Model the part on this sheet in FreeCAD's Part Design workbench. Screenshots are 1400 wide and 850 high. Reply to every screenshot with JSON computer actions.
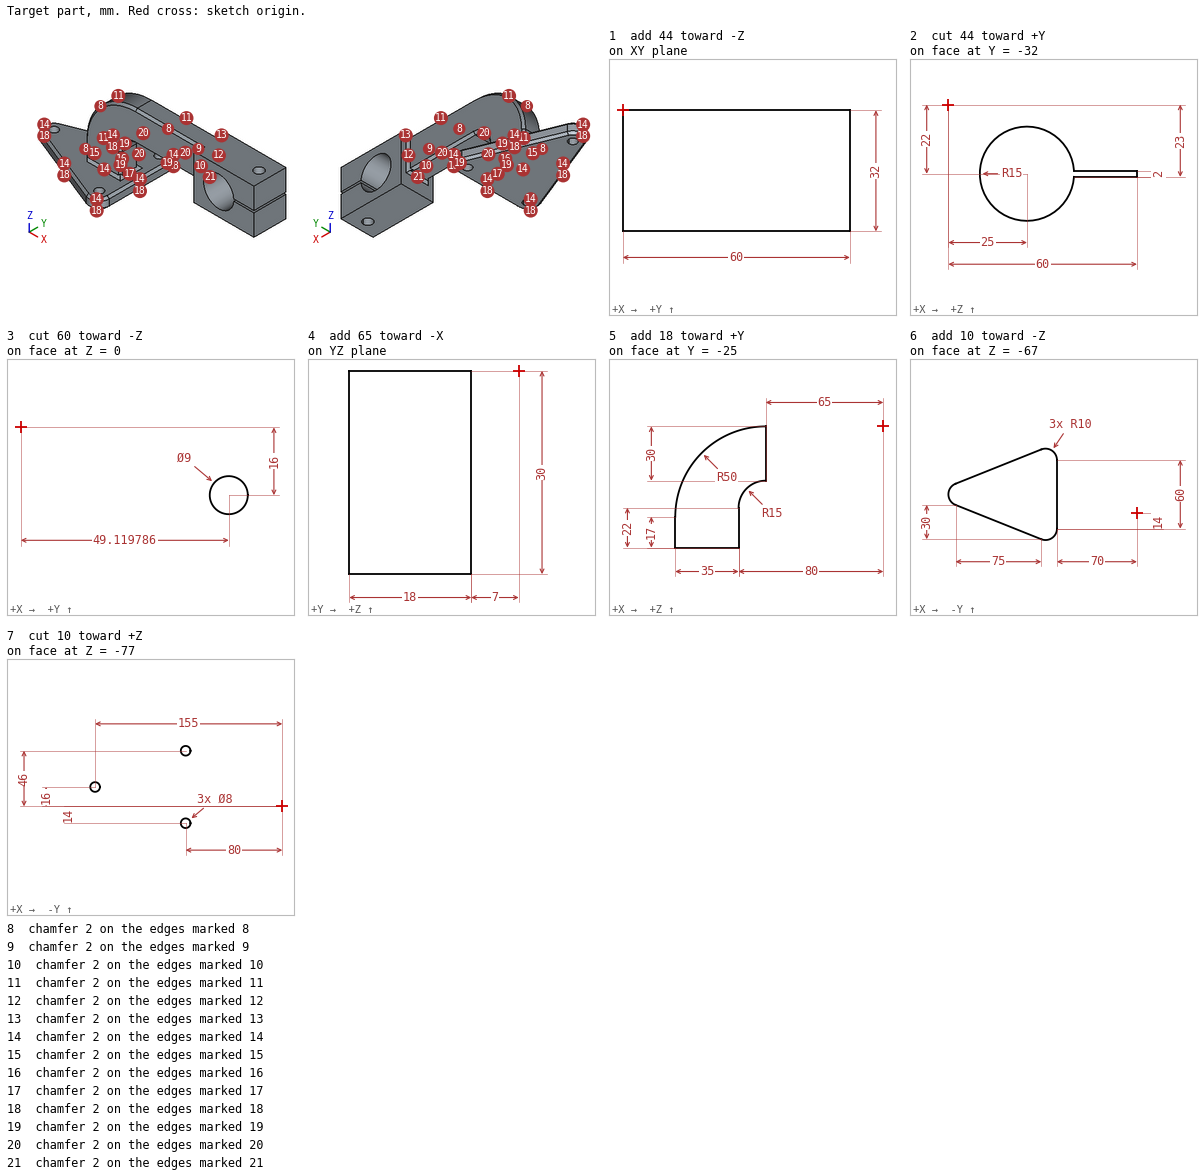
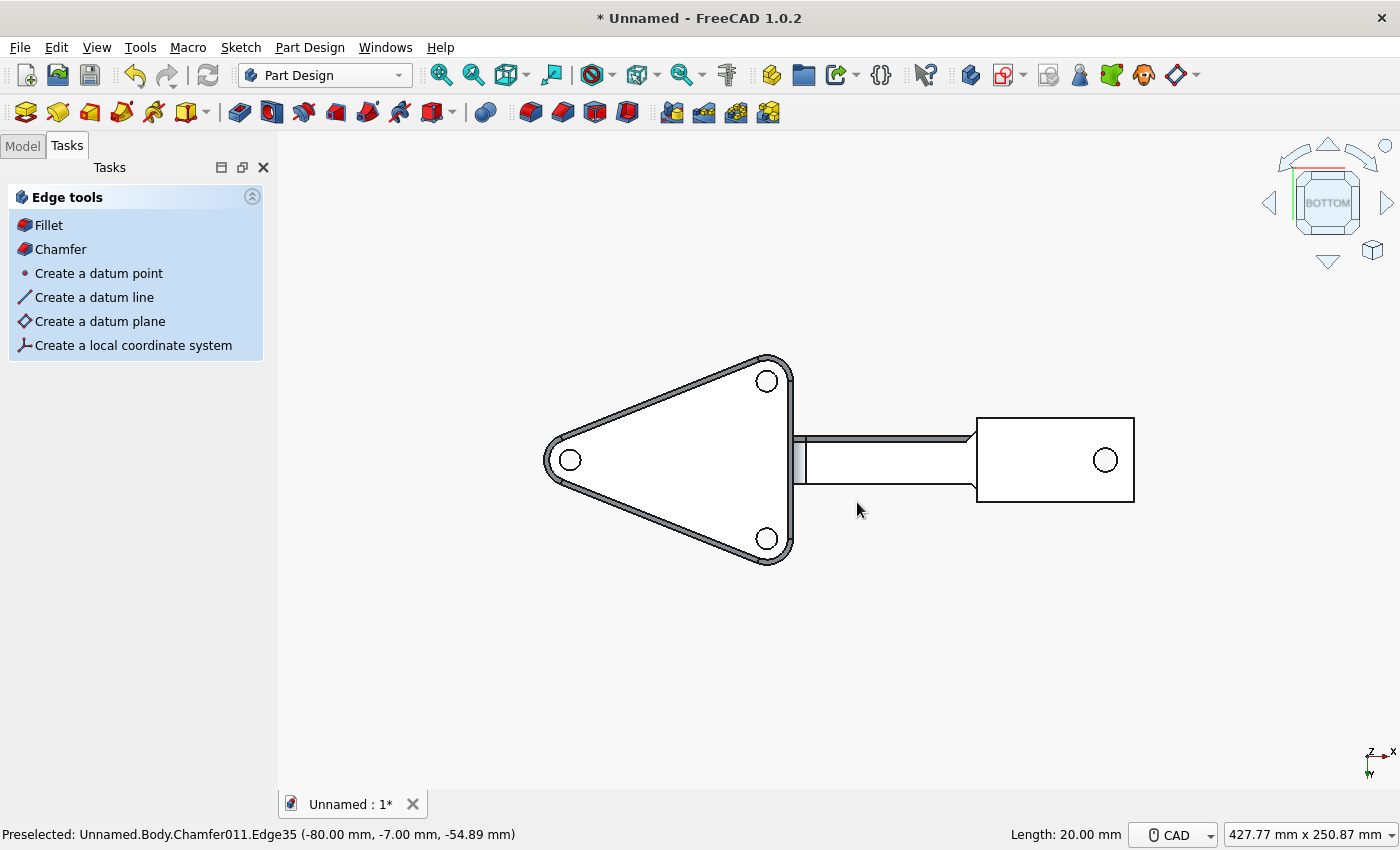
{"action": "left_click", "coordinate": [889, 483], "text": "ctrl"}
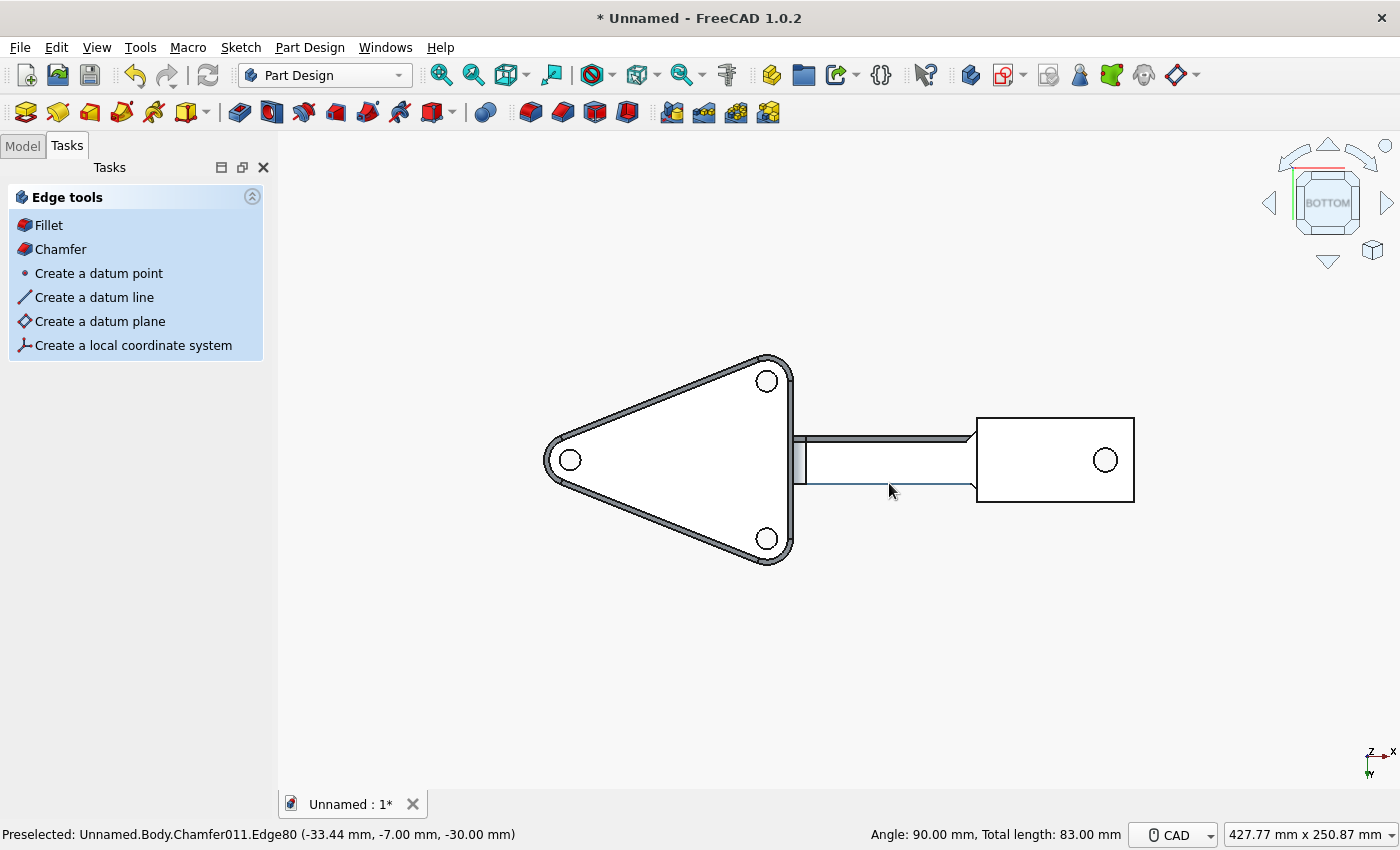
{"action": "left_click", "coordinate": [804, 483], "text": "ctrl"}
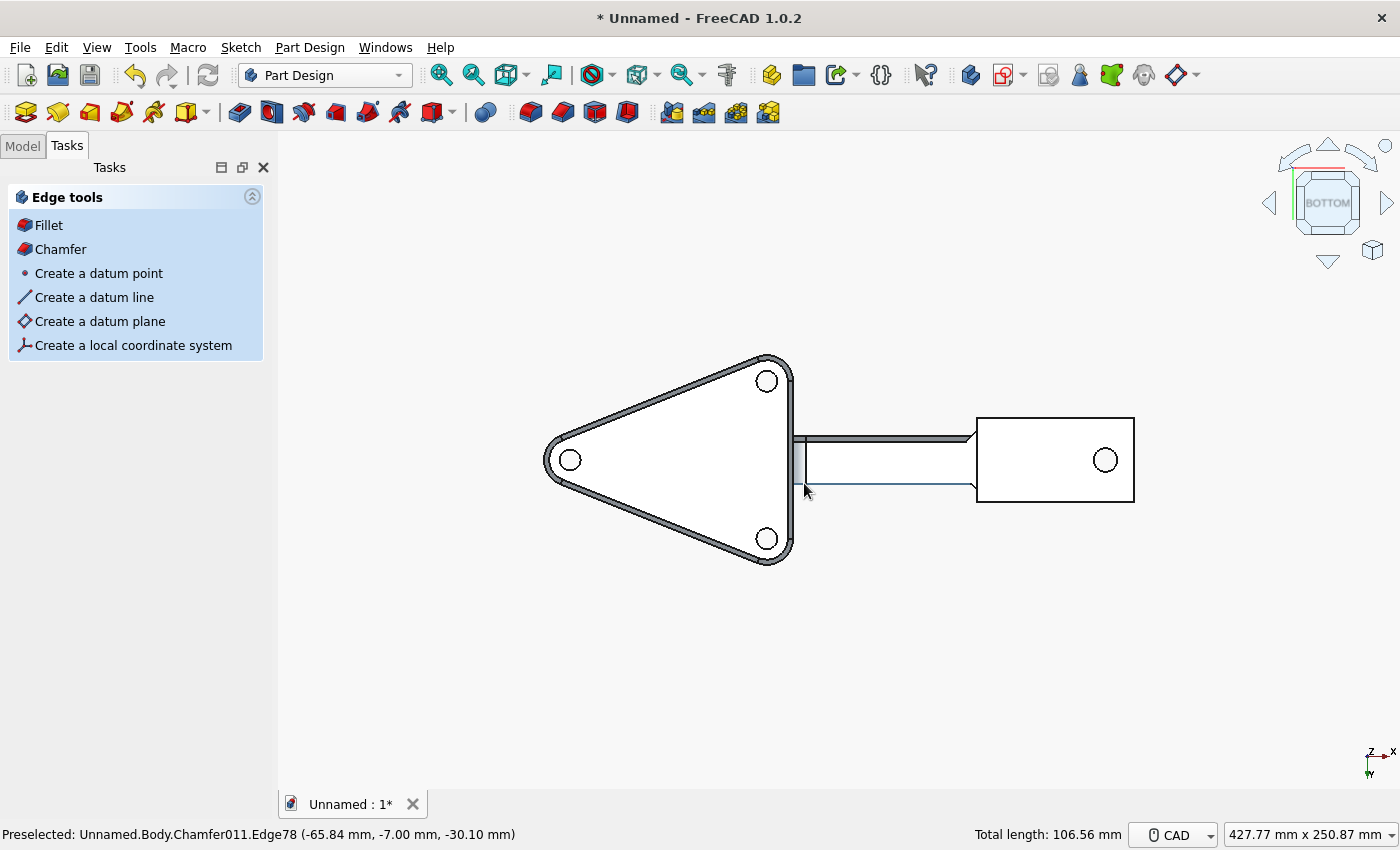
{"action": "left_click", "coordinate": [564, 112]}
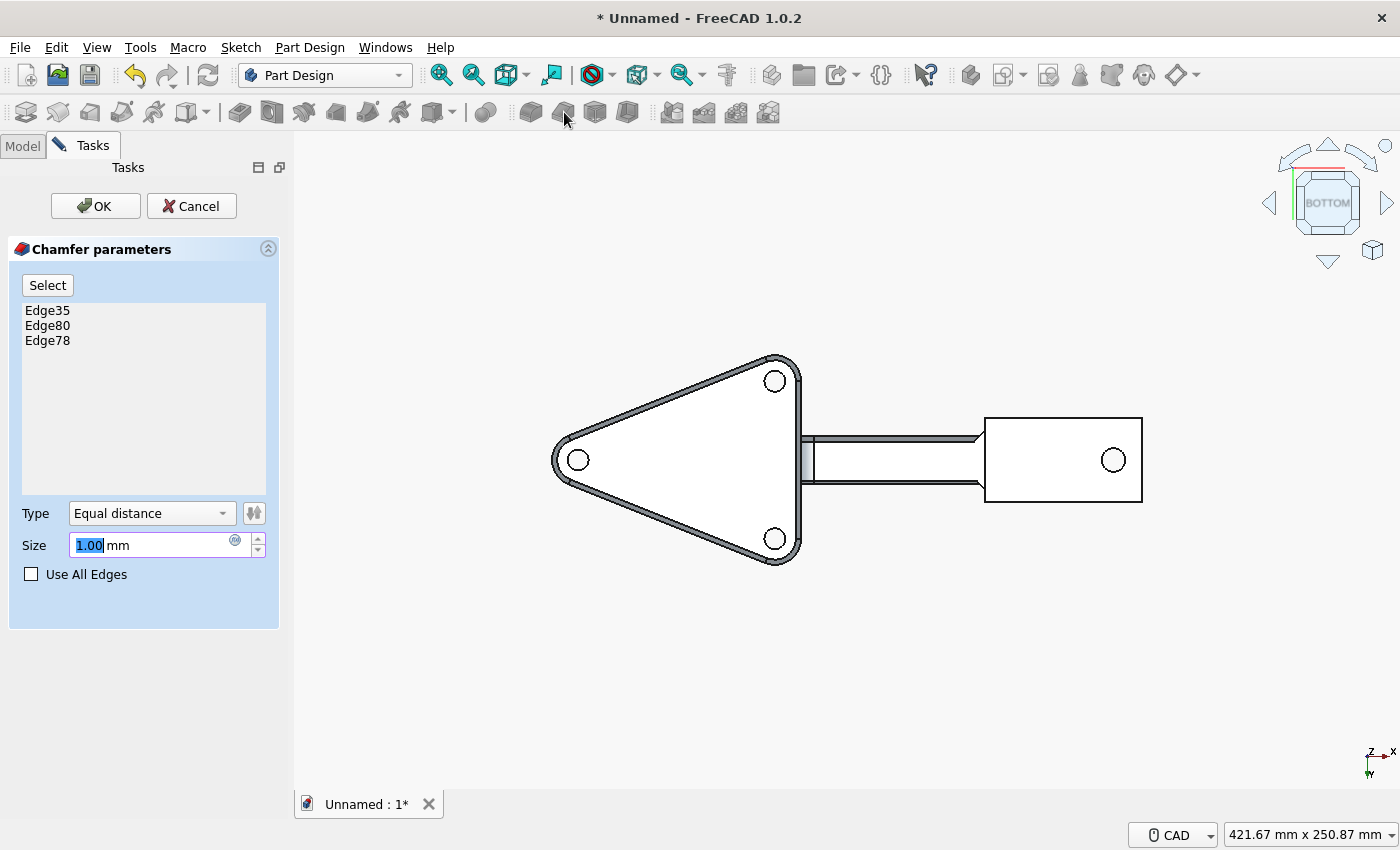
{"action": "type", "text": "2"}
{"action": "key", "text": "Tab"}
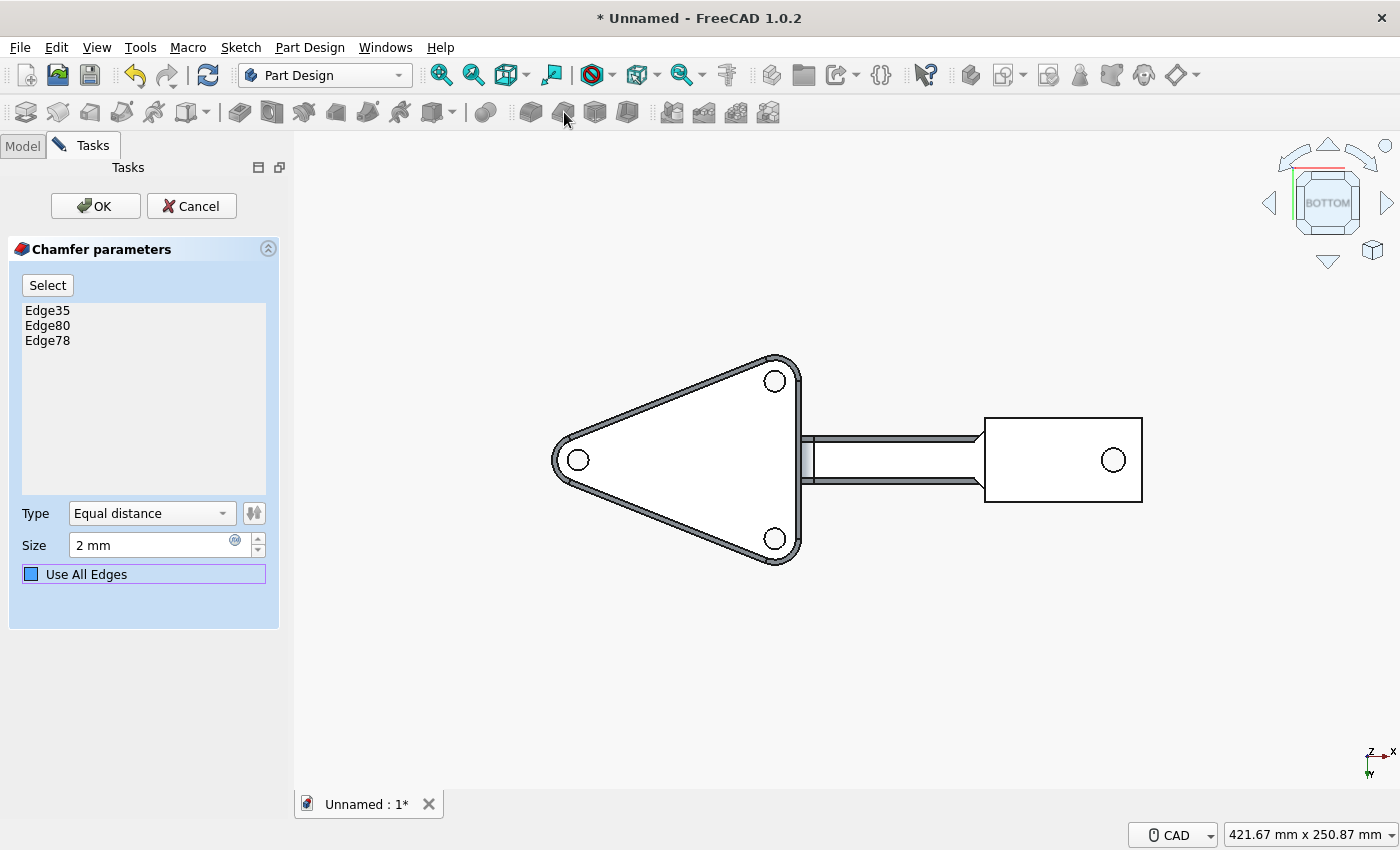
{"action": "left_click", "coordinate": [96, 206]}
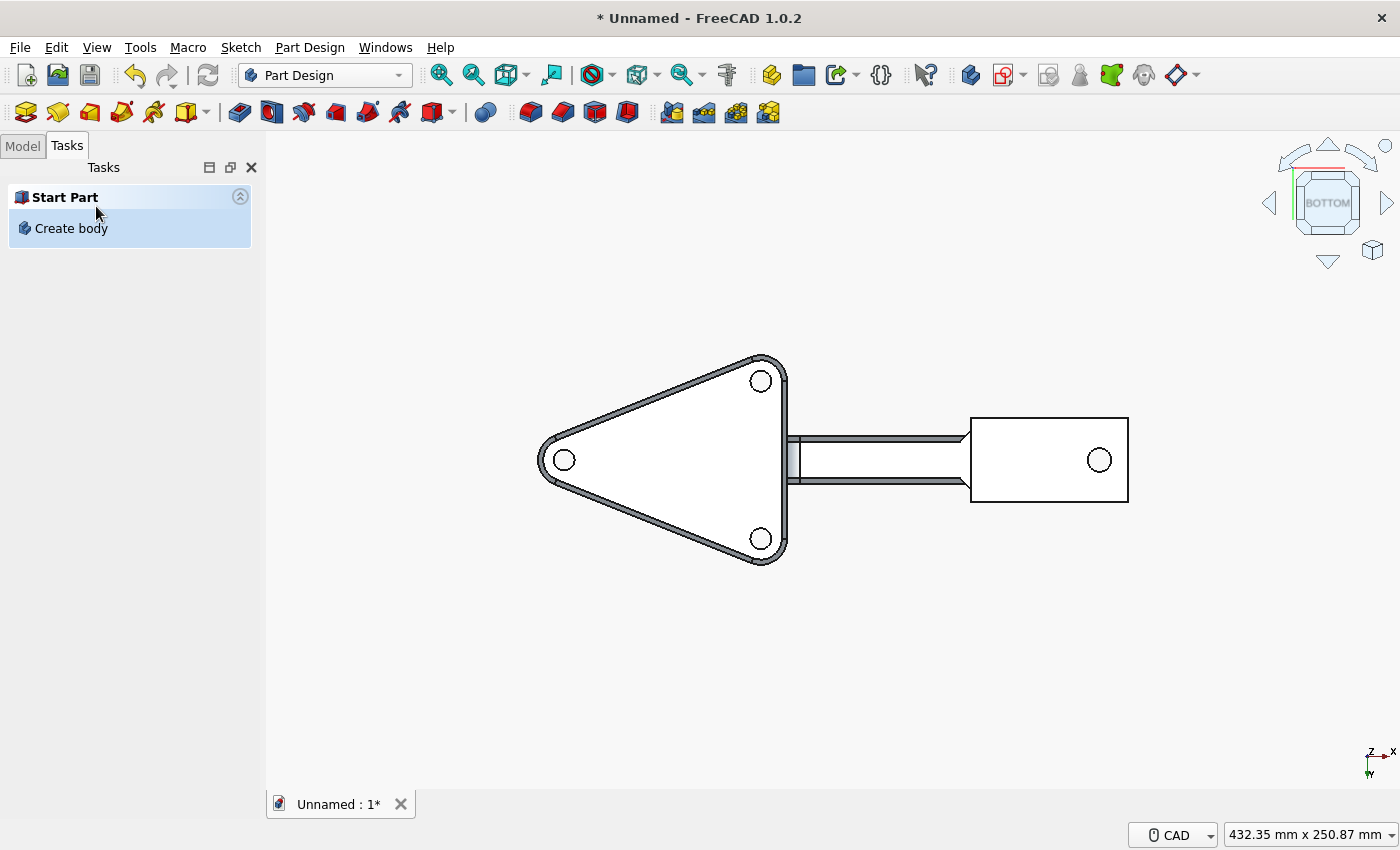
{"action": "key", "text": "0"}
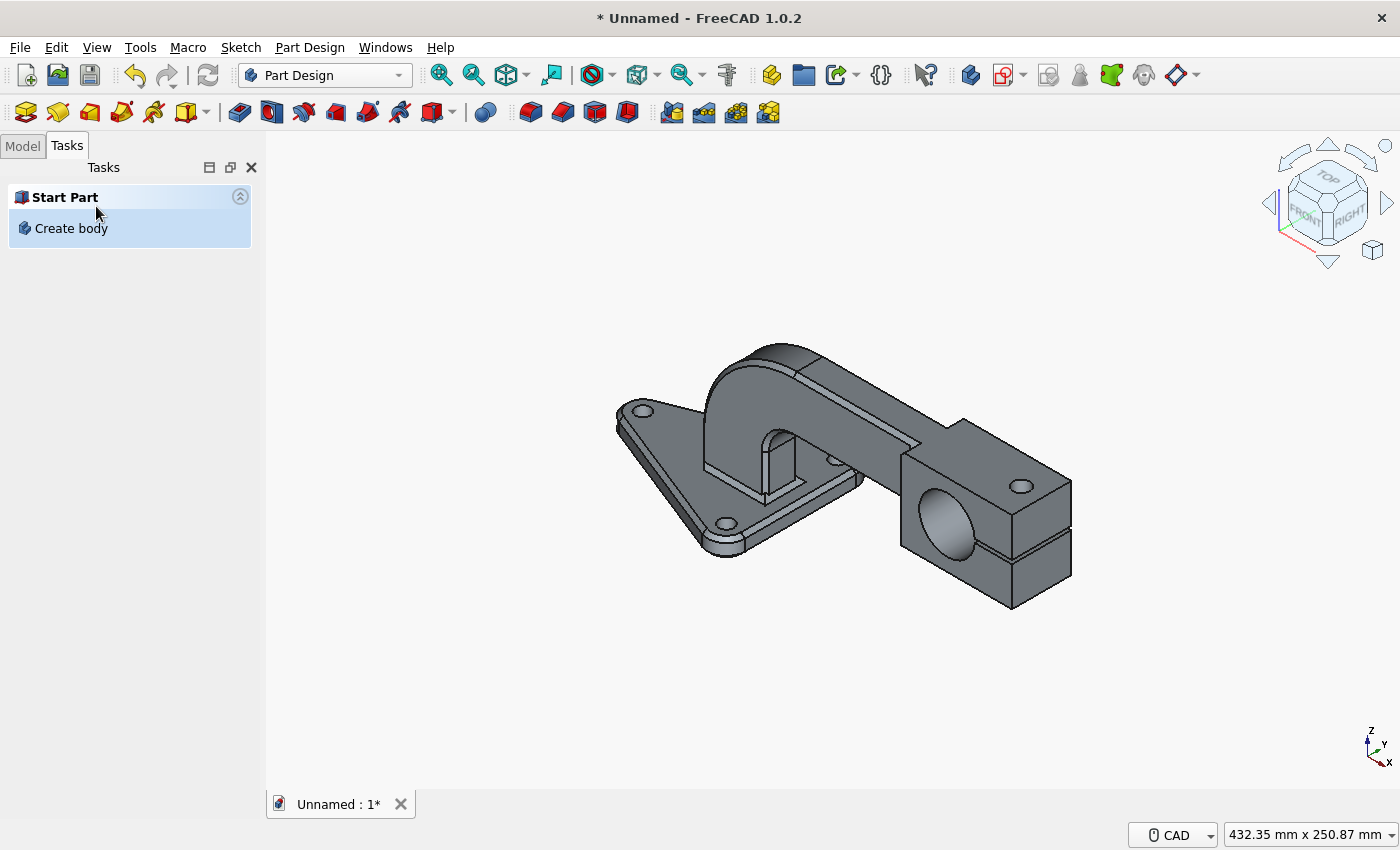
{"action": "key", "text": "2"}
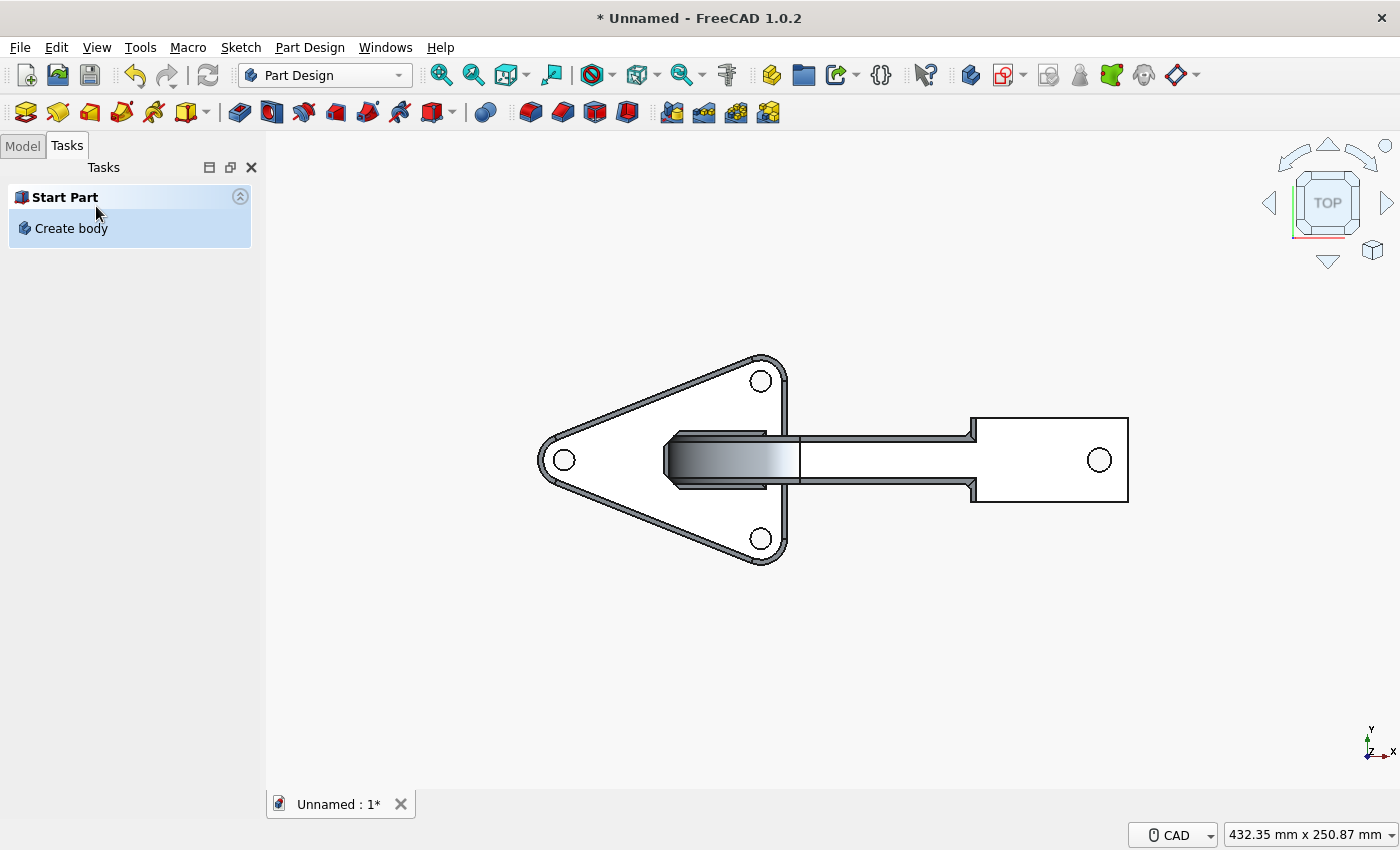
{"action": "key", "text": "1"}